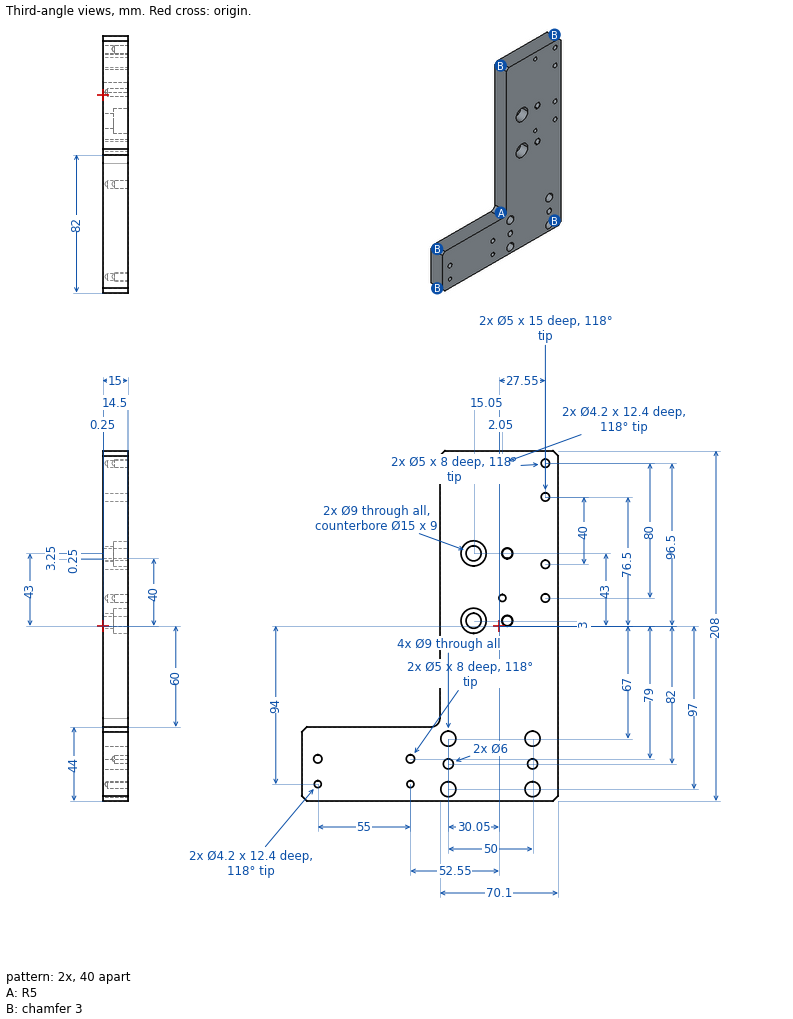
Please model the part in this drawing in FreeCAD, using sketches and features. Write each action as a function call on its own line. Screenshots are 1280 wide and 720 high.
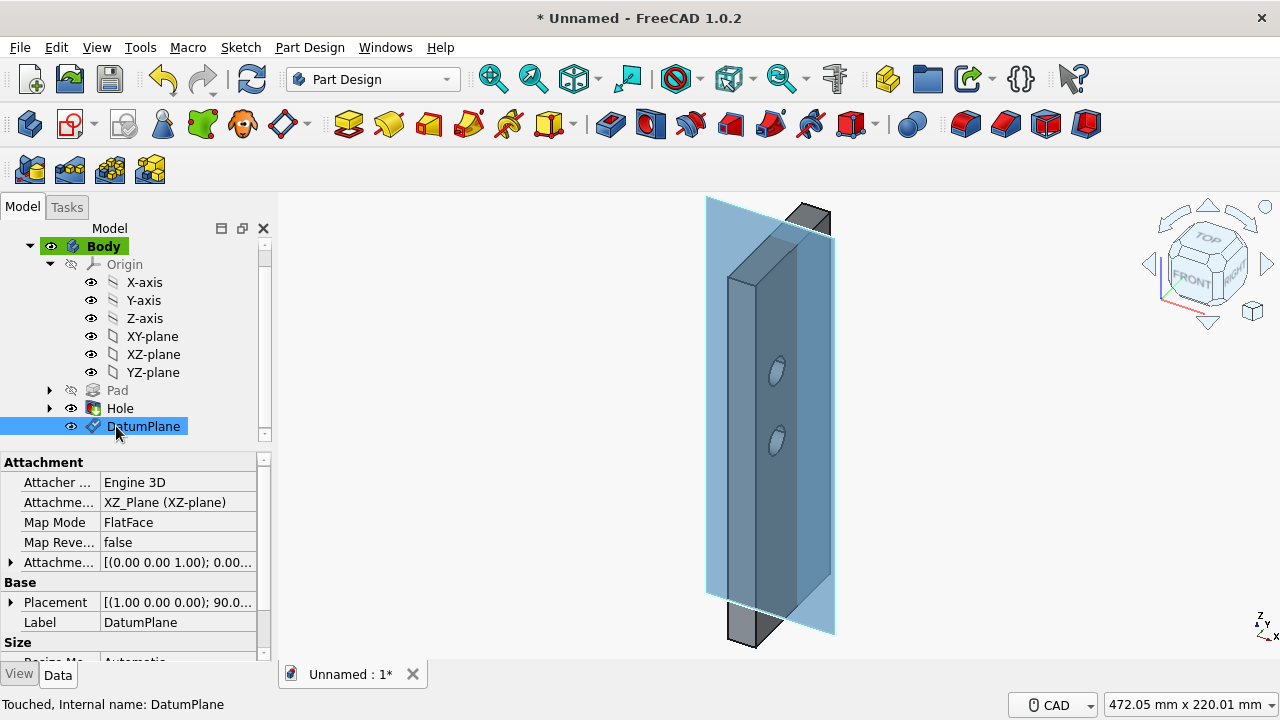
click(70, 124)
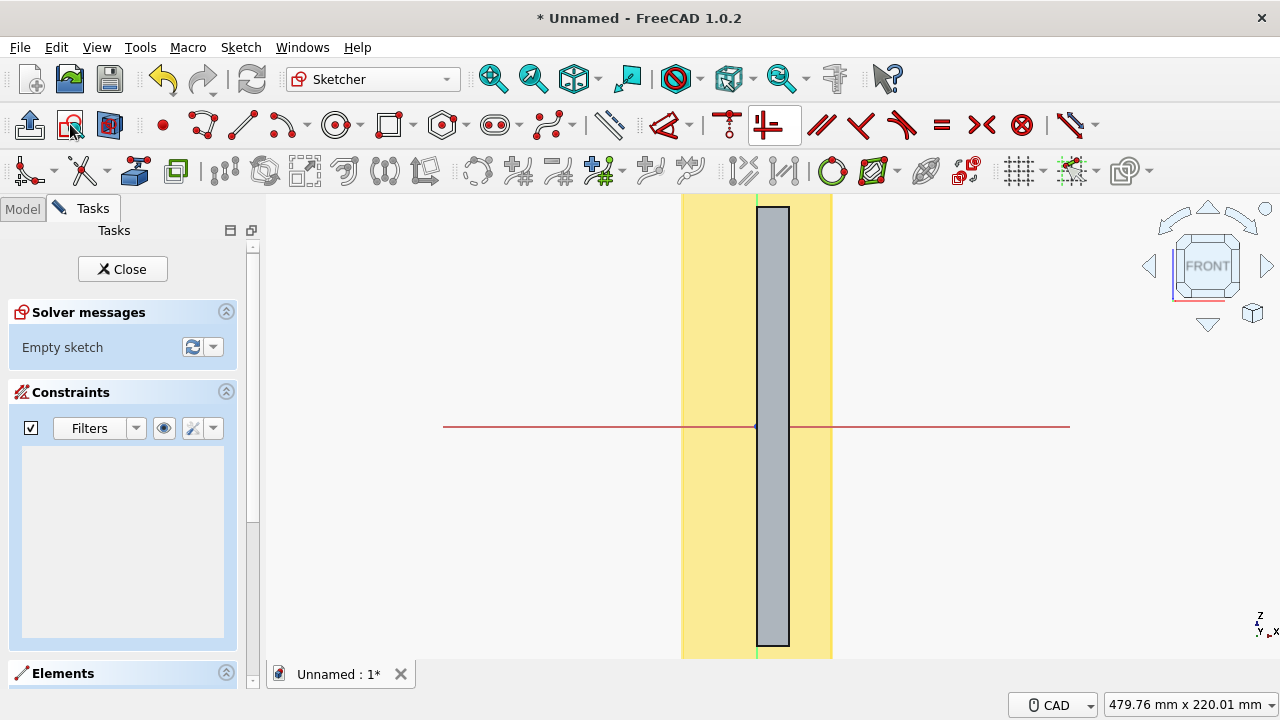
click(110, 126)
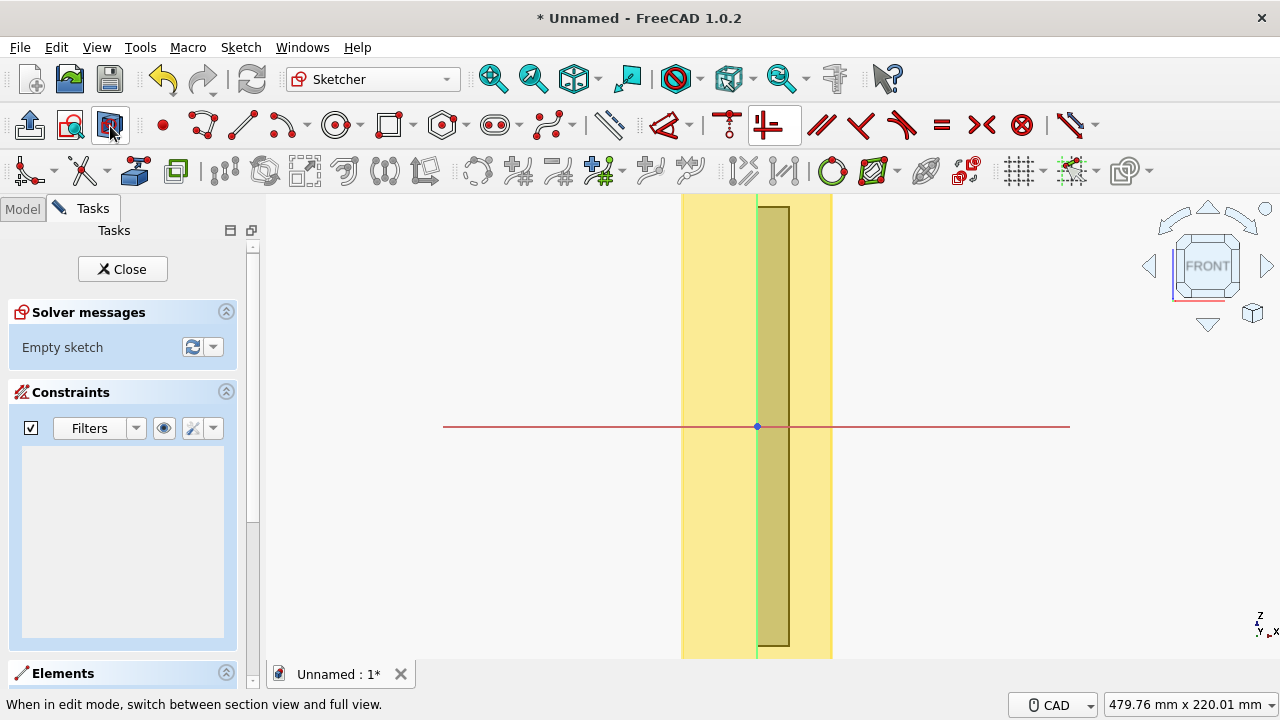
scroll(793, 361, up, 6)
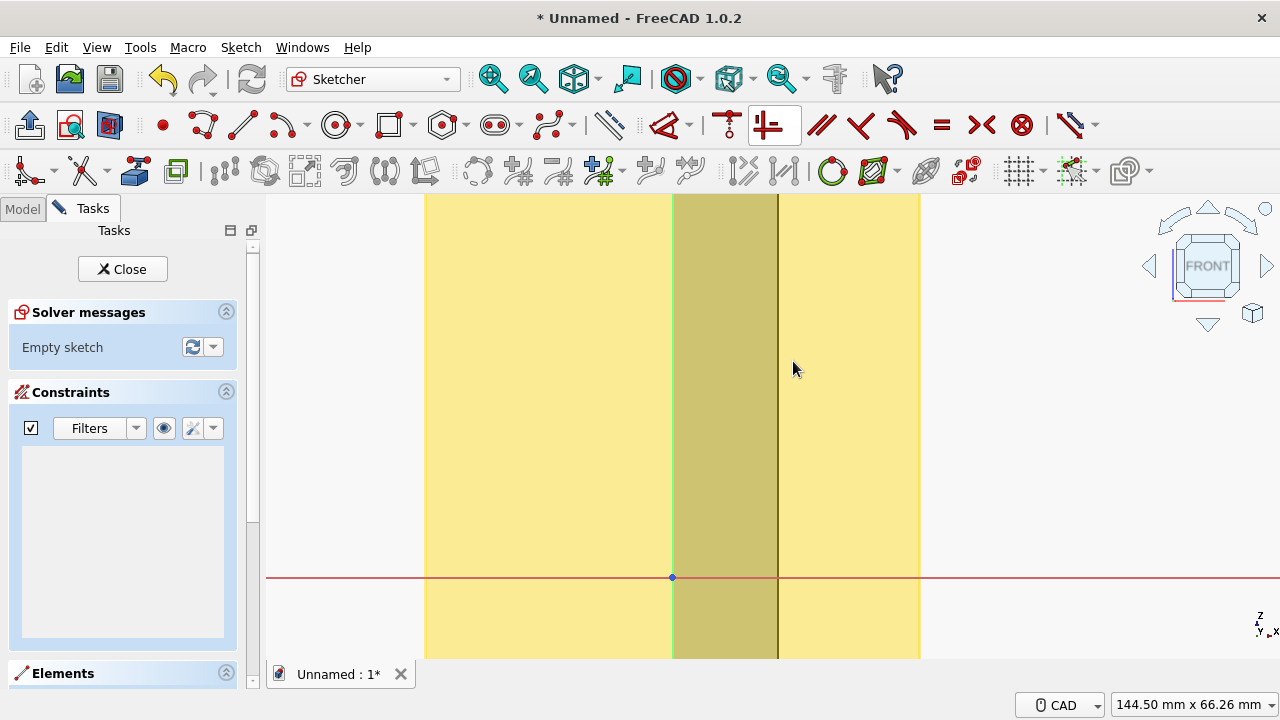
click(204, 126)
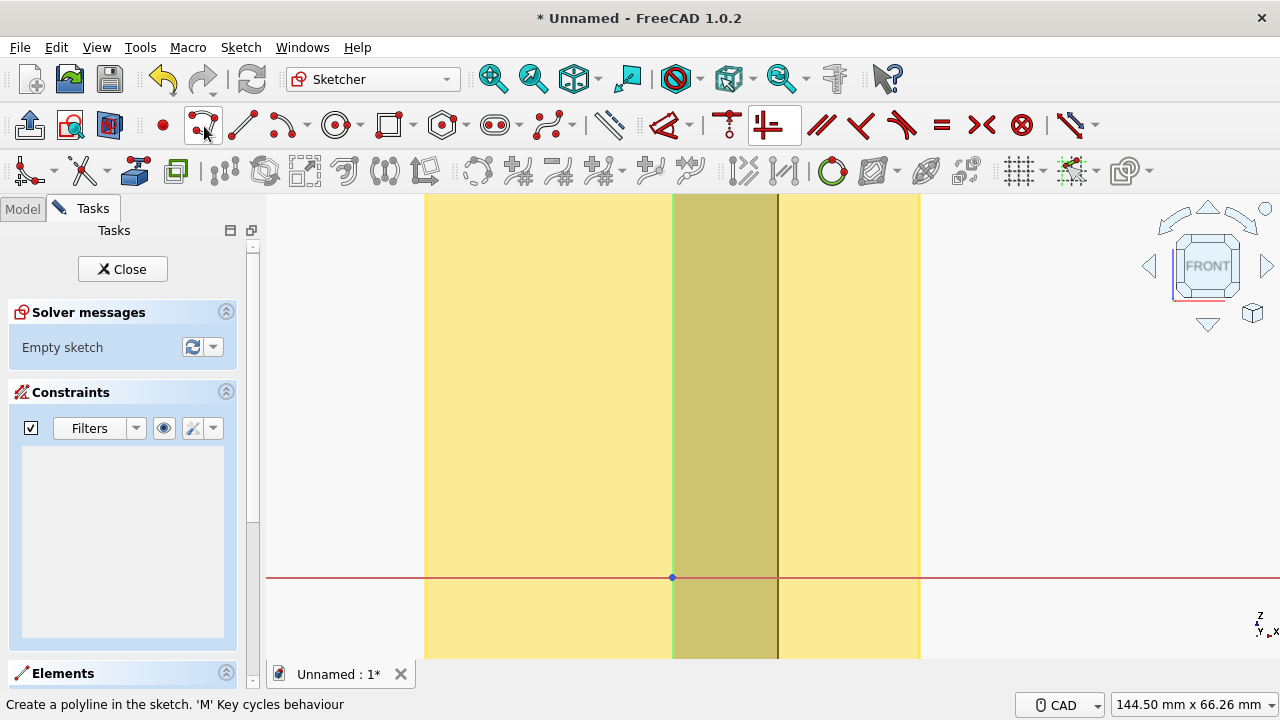
click(673, 299)
click(682, 276)
click(778, 276)
click(778, 299)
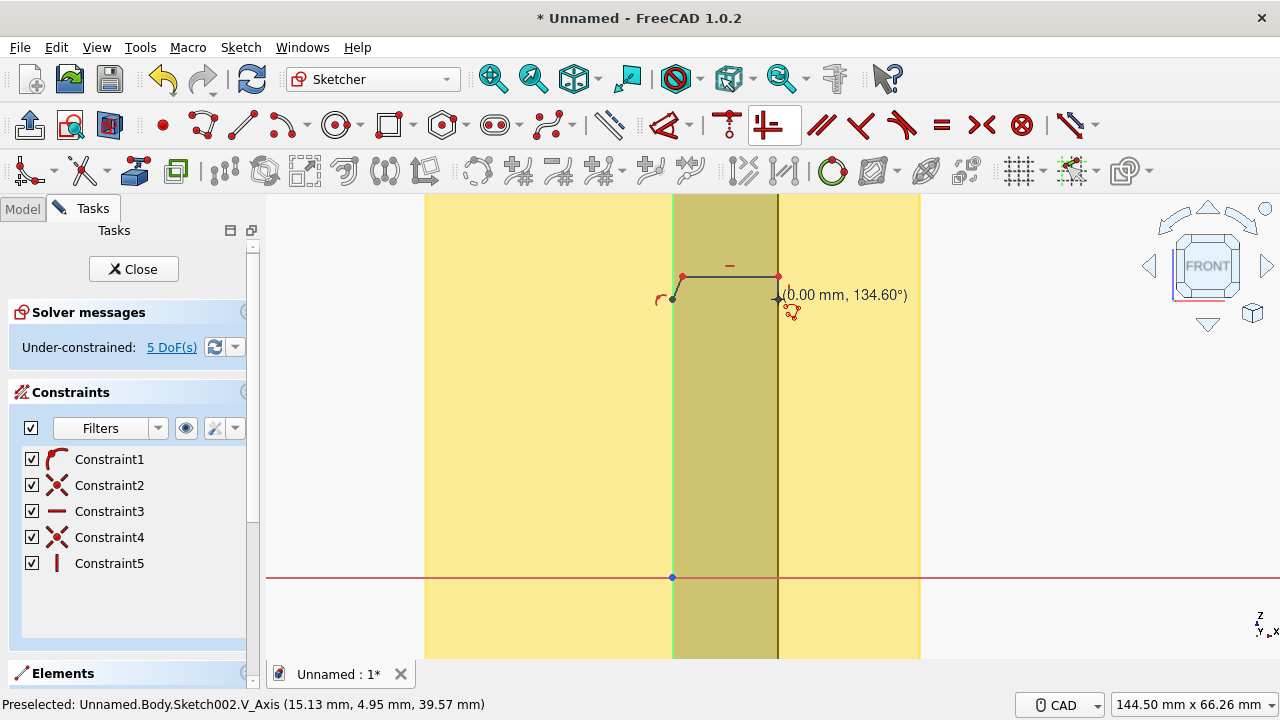
scroll(776, 297, up, 12)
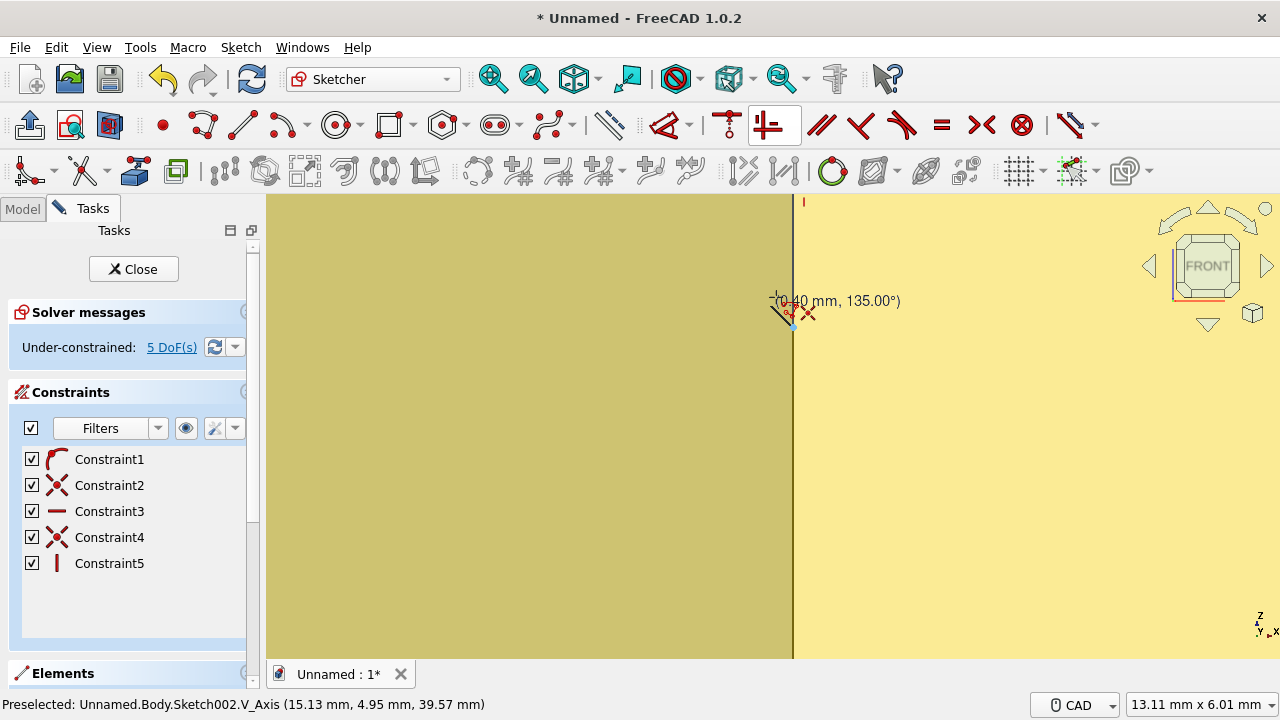
click(774, 294)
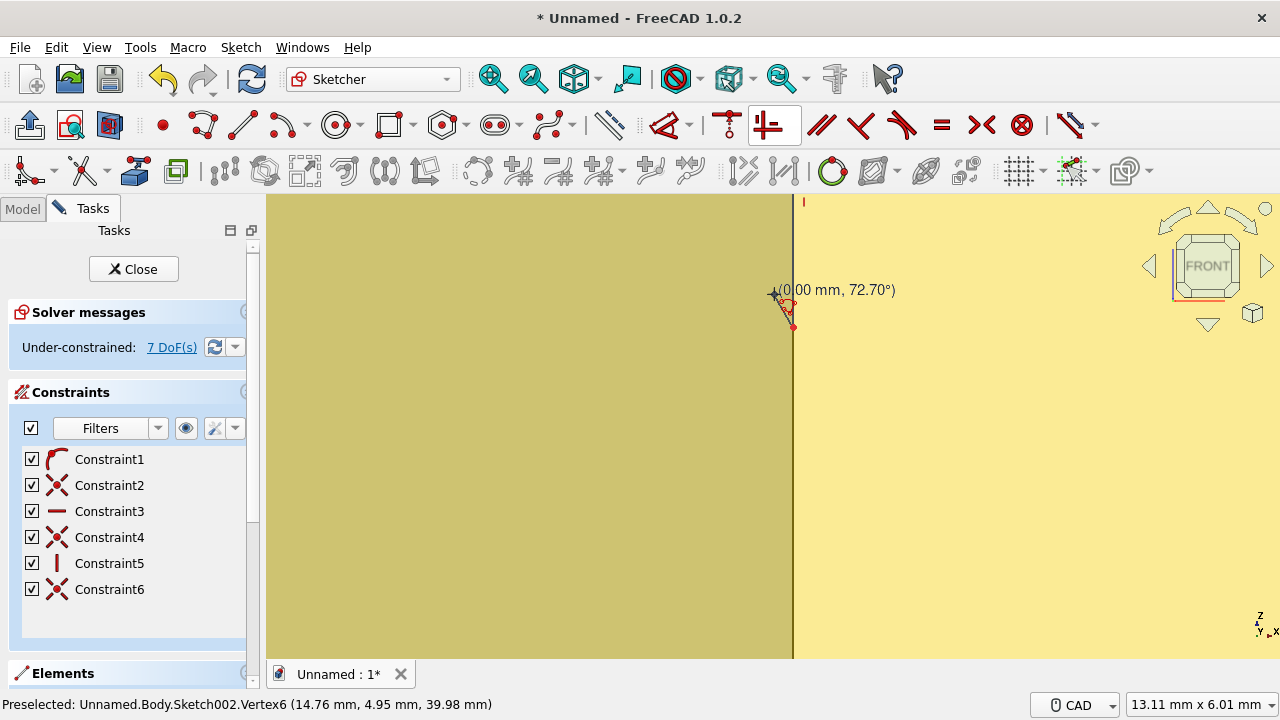
scroll(777, 297, down, 12)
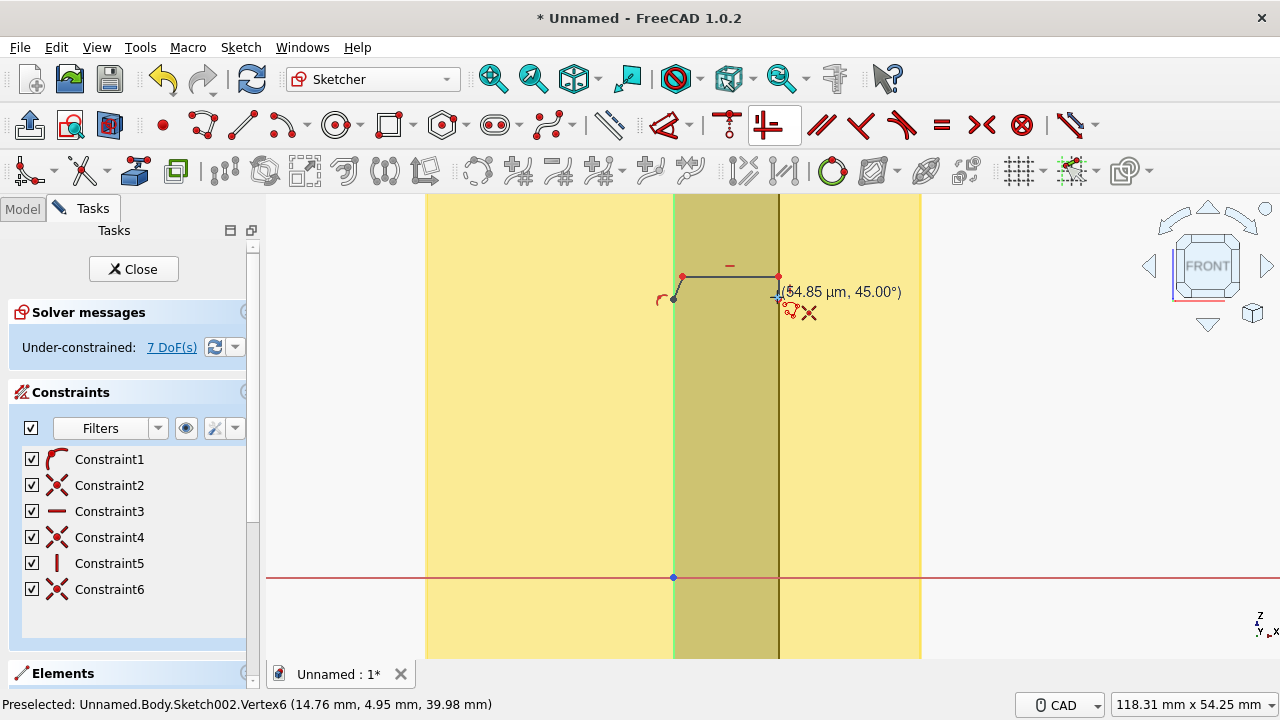
scroll(675, 297, up, 12)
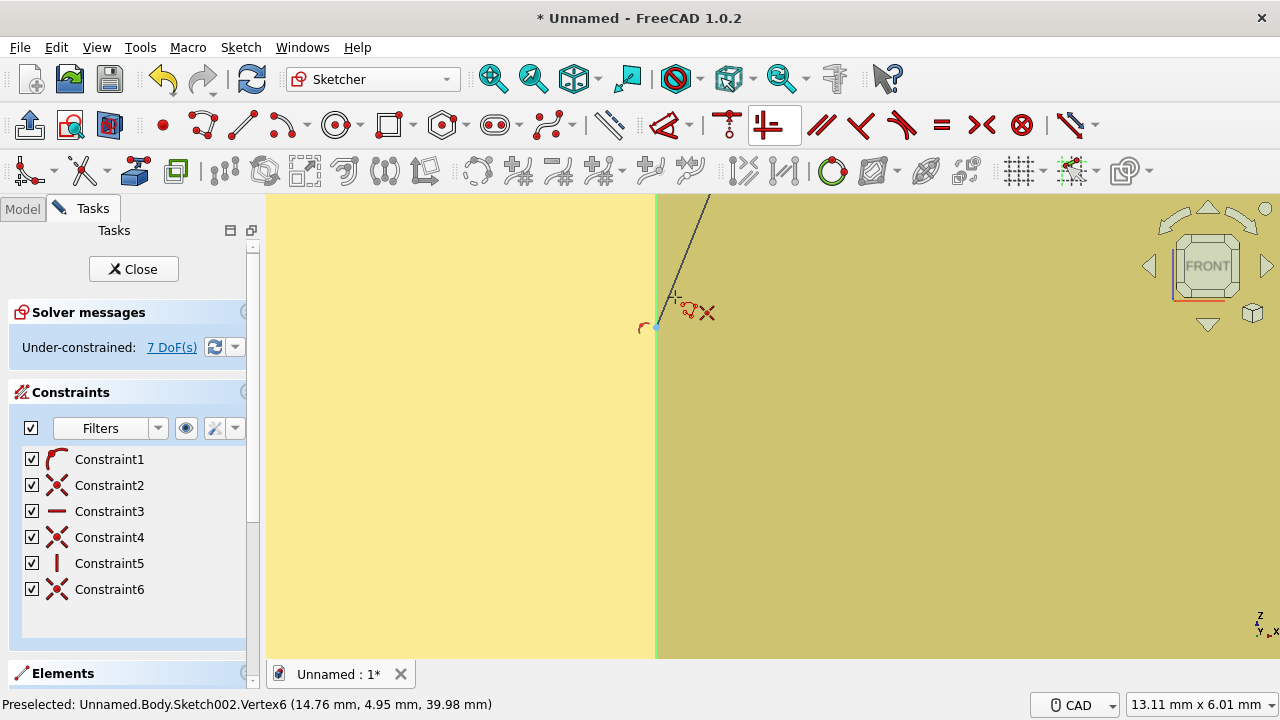
click(676, 294)
click(656, 317)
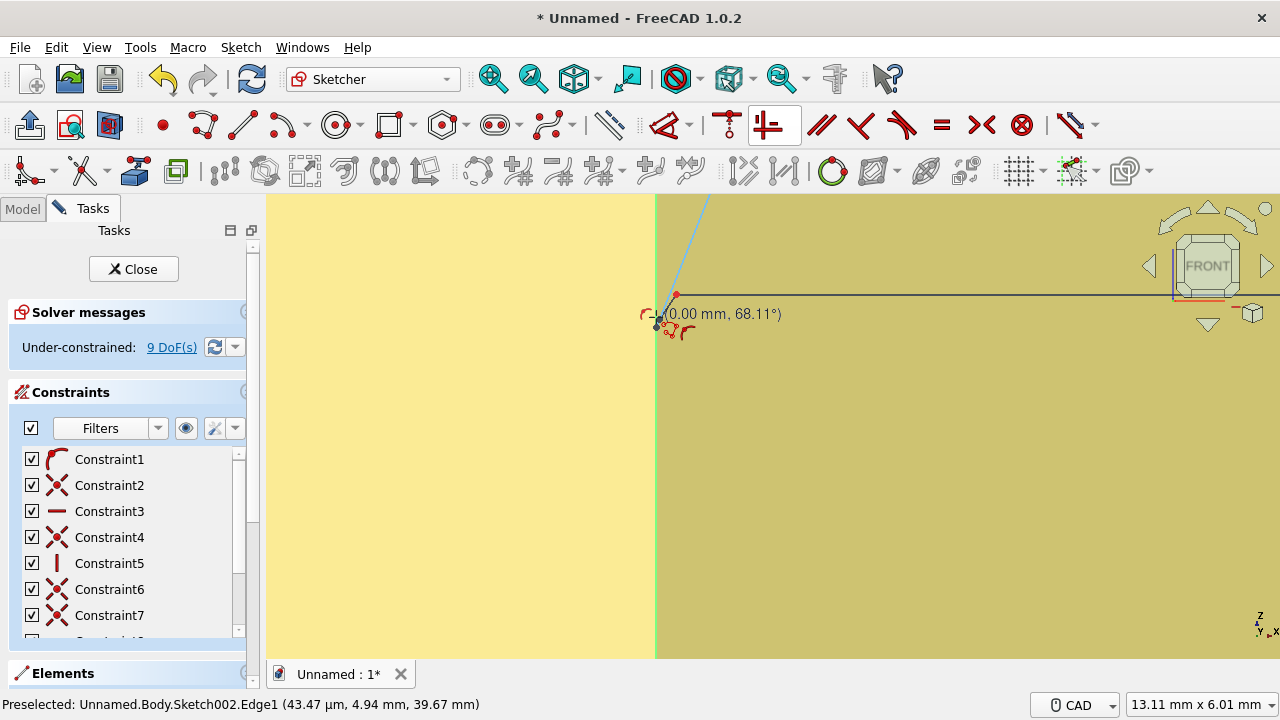
click(244, 126)